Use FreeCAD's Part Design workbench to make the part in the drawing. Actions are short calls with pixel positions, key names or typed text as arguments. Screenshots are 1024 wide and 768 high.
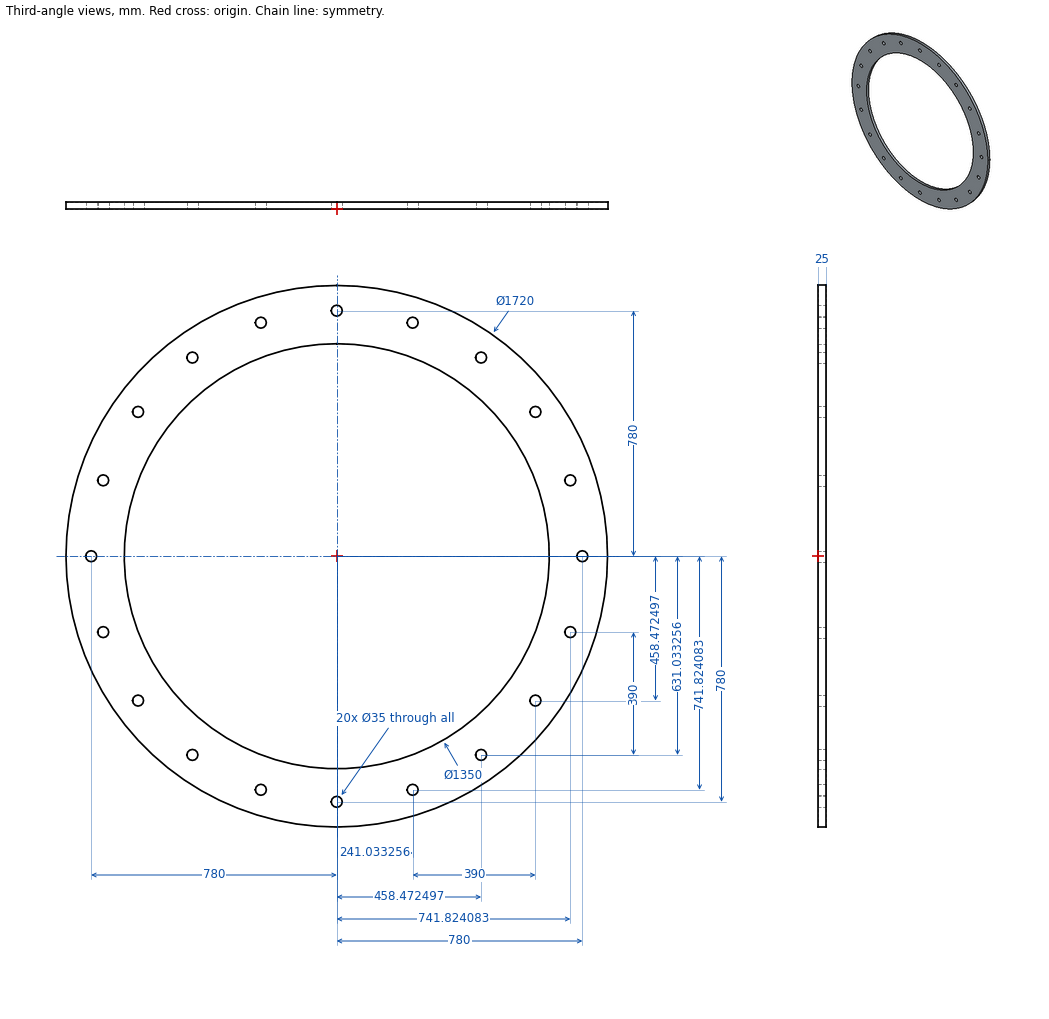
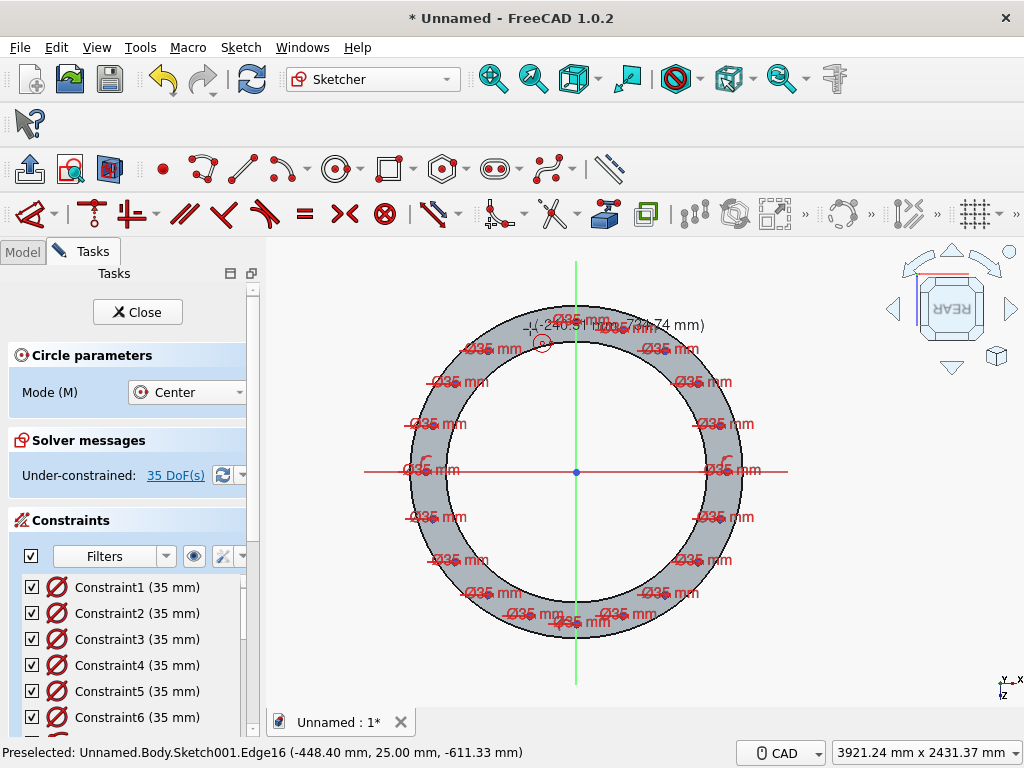
click(530, 329)
move(532, 326)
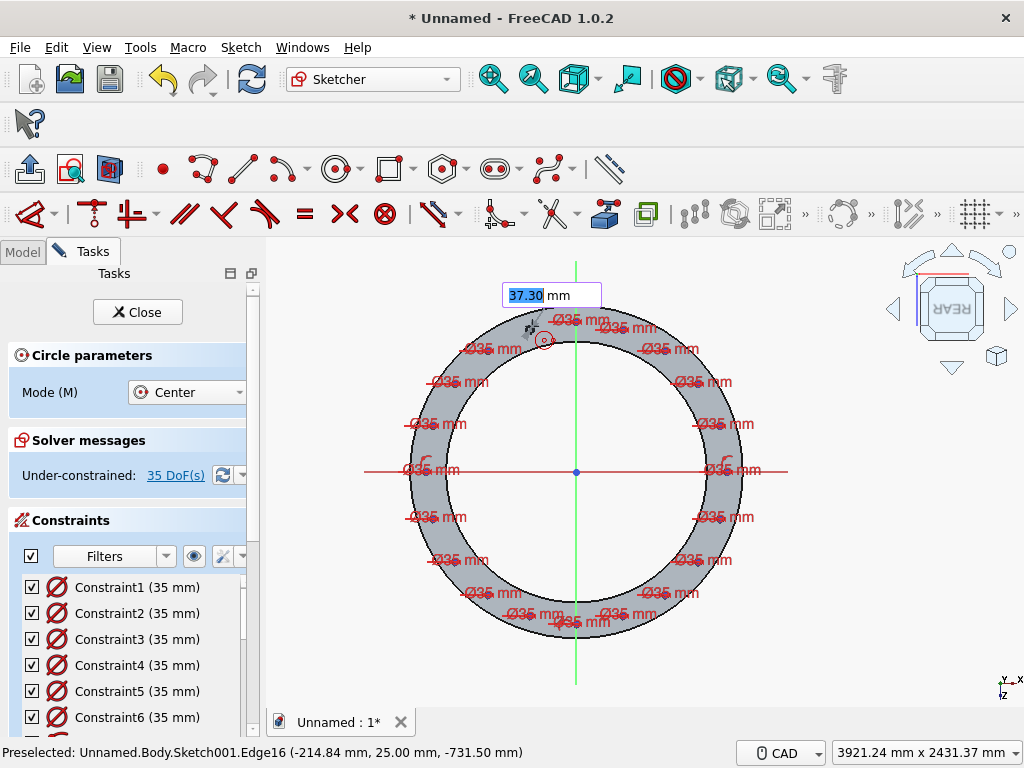
text(35)
key(Return)
key(Escape)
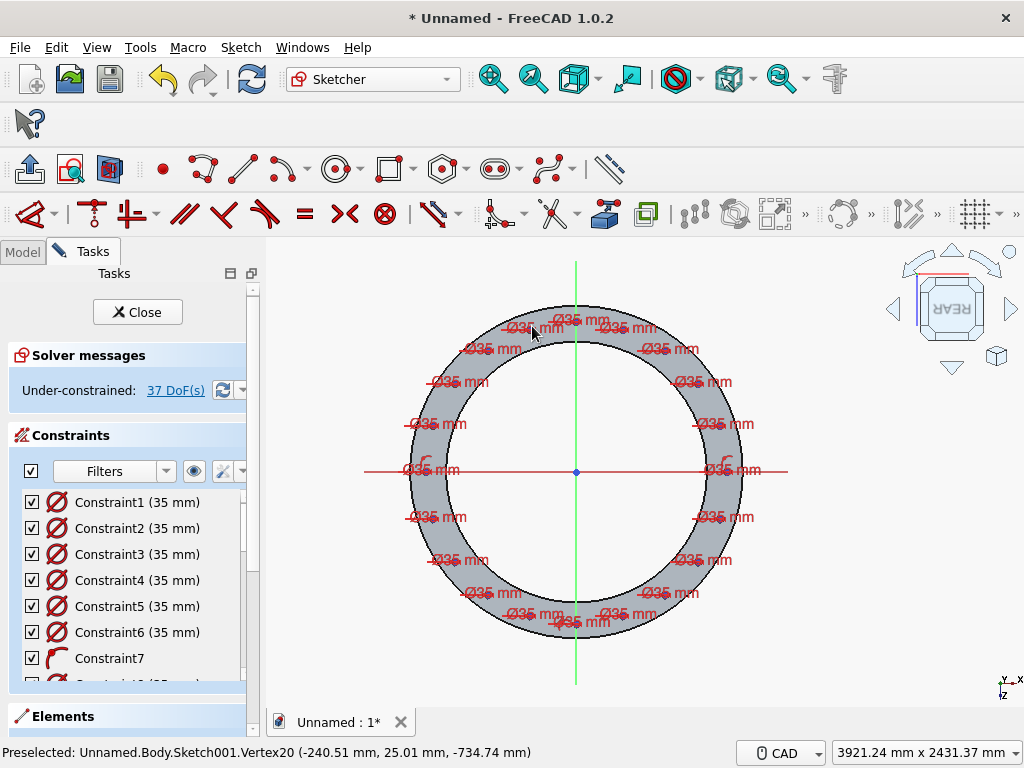
click(576, 322)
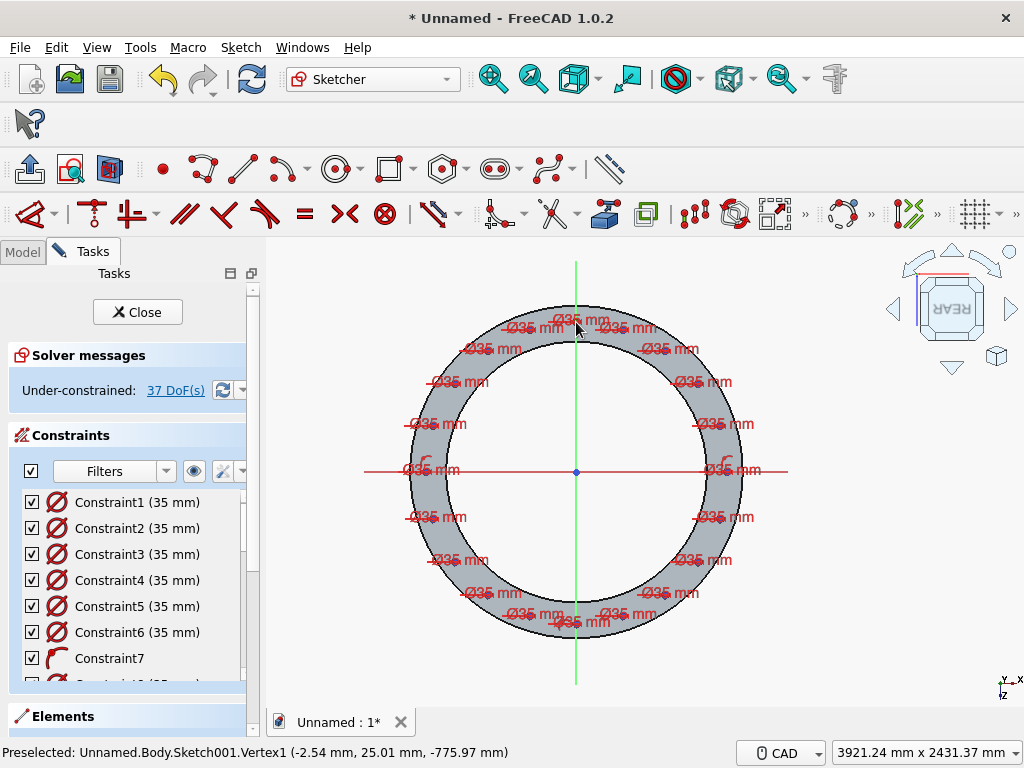
click(576, 590)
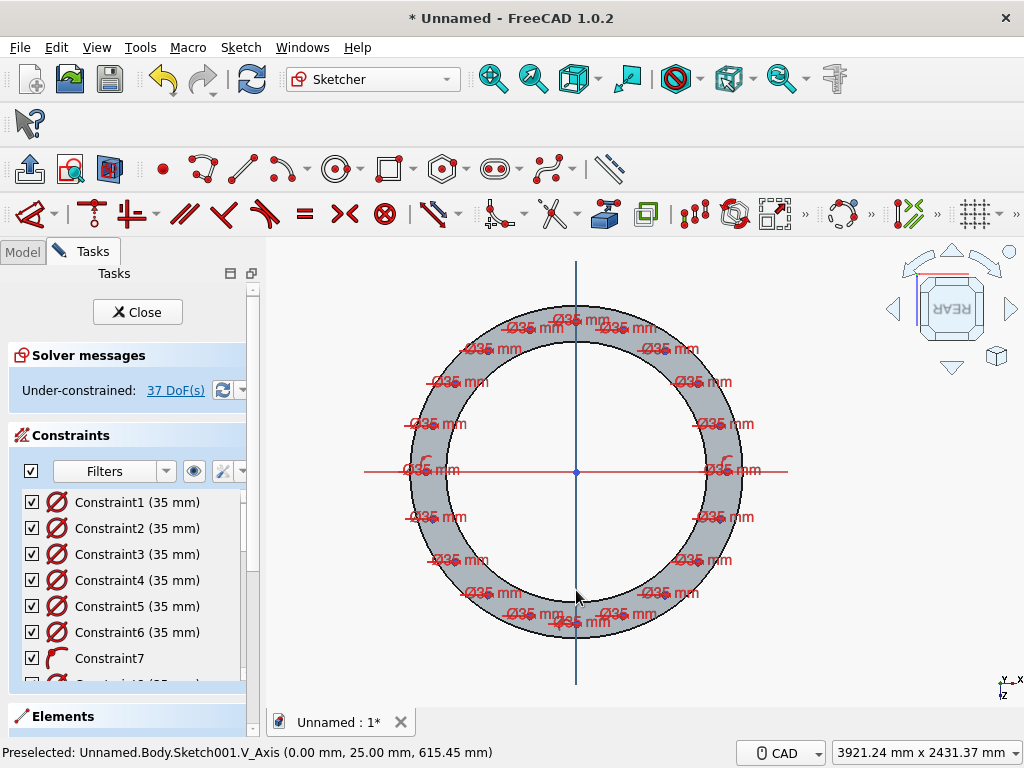
key(c)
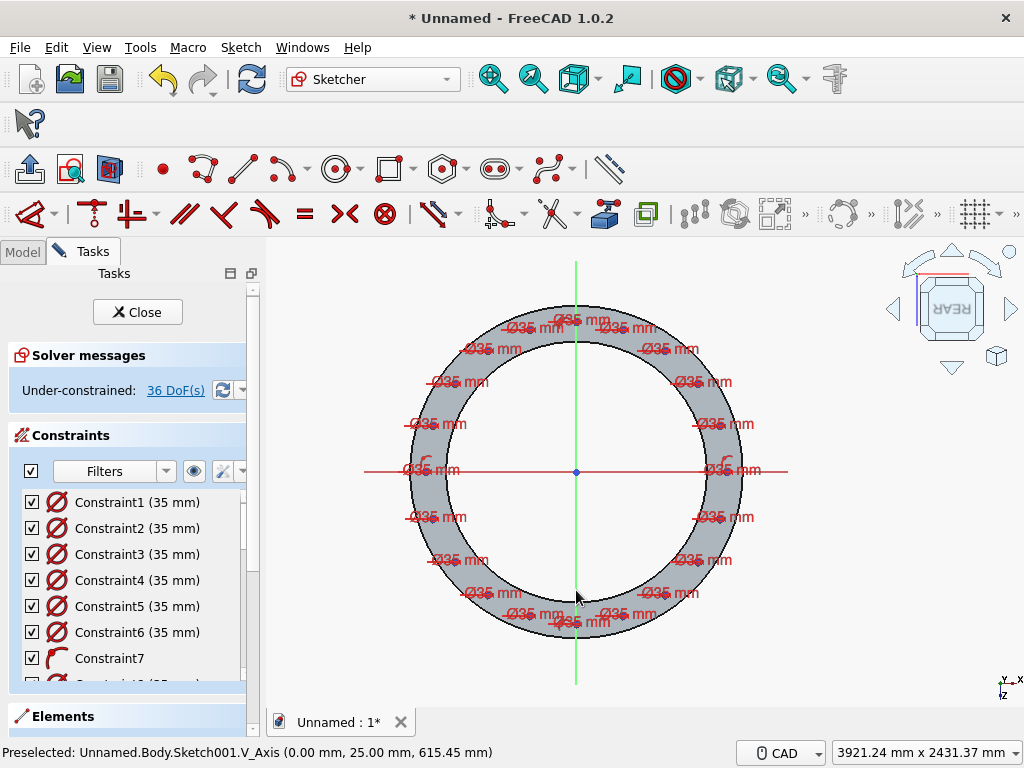
click(720, 426)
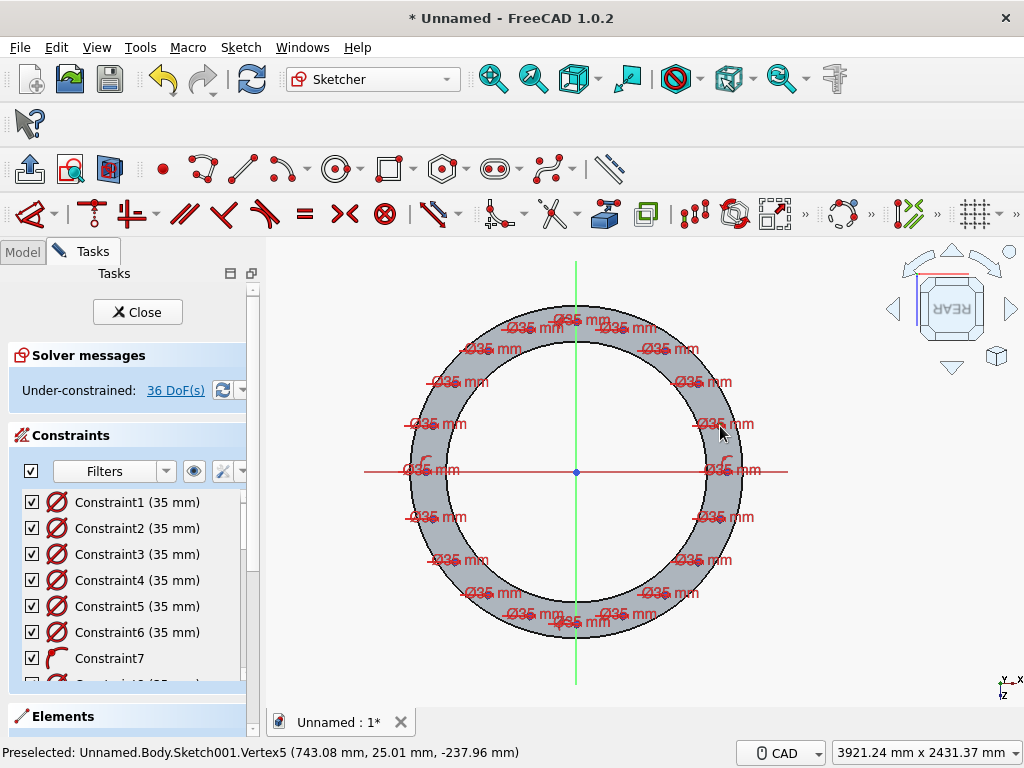
click(720, 519)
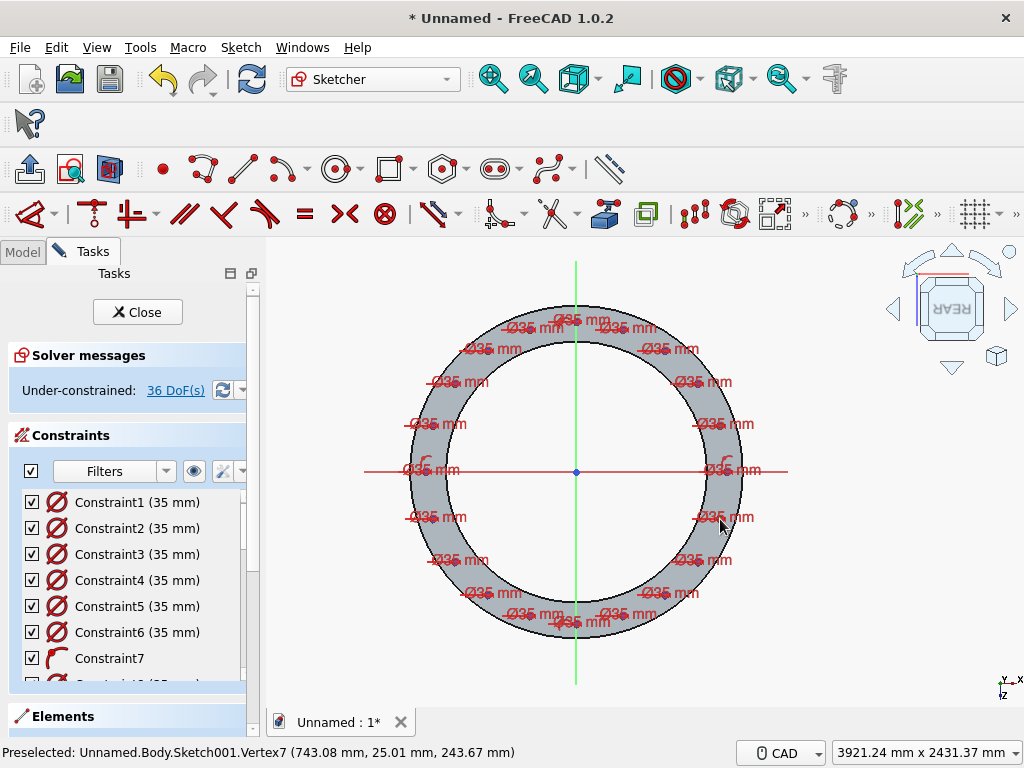
click(375, 472)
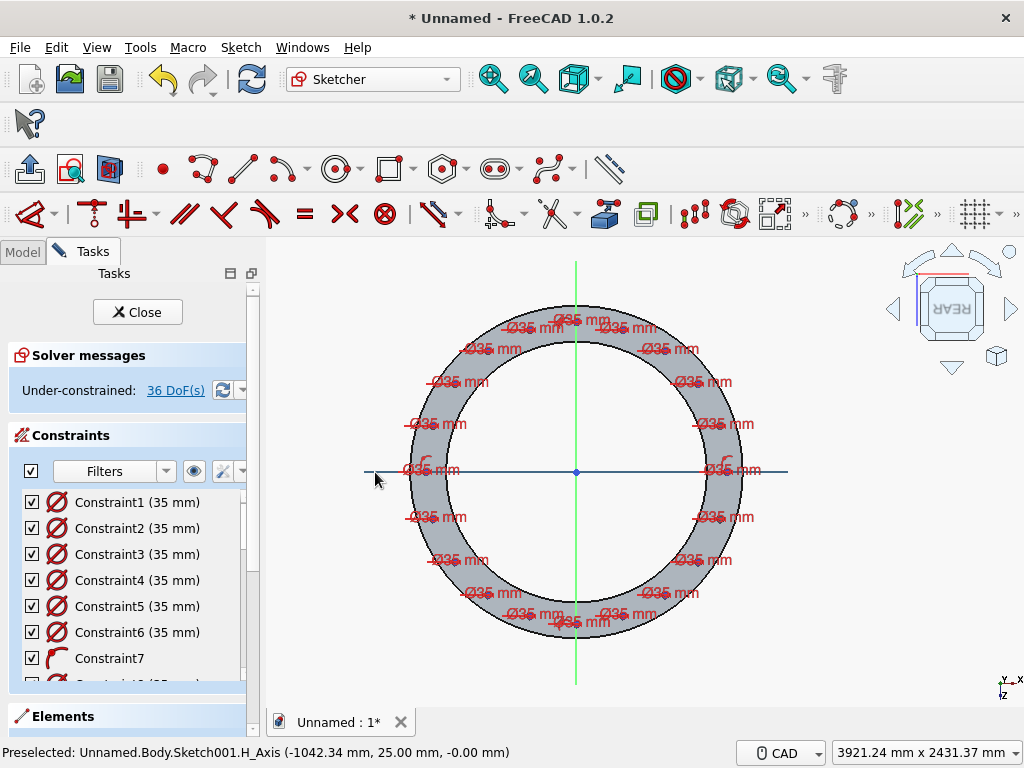
click(346, 214)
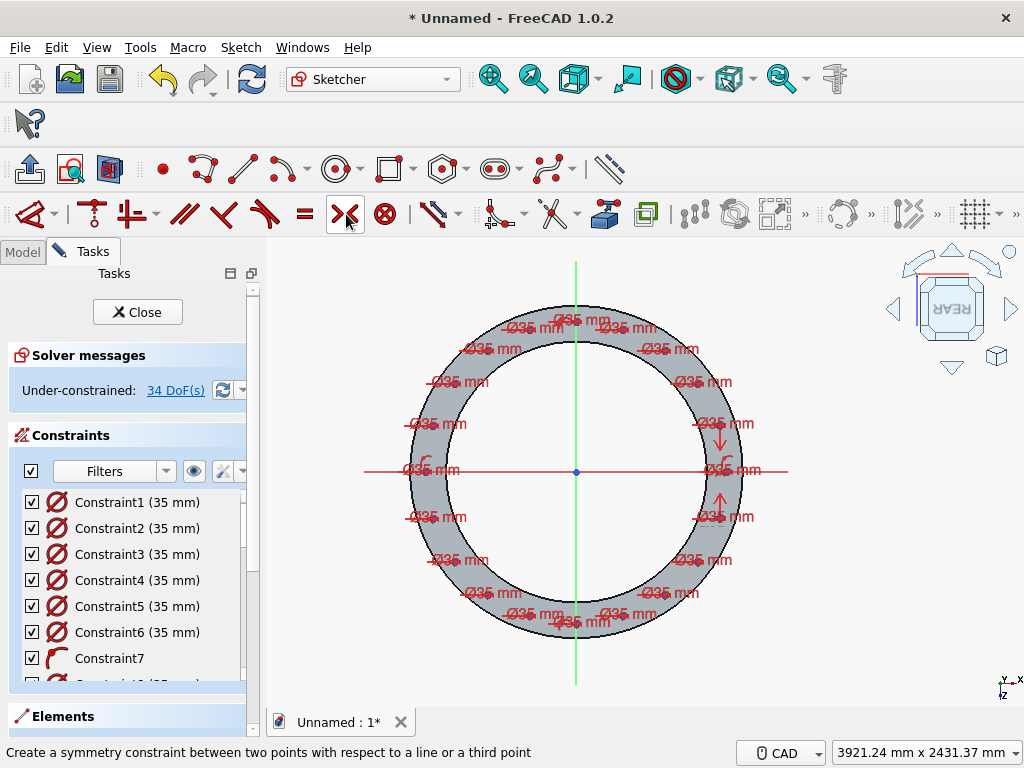
click(698, 384)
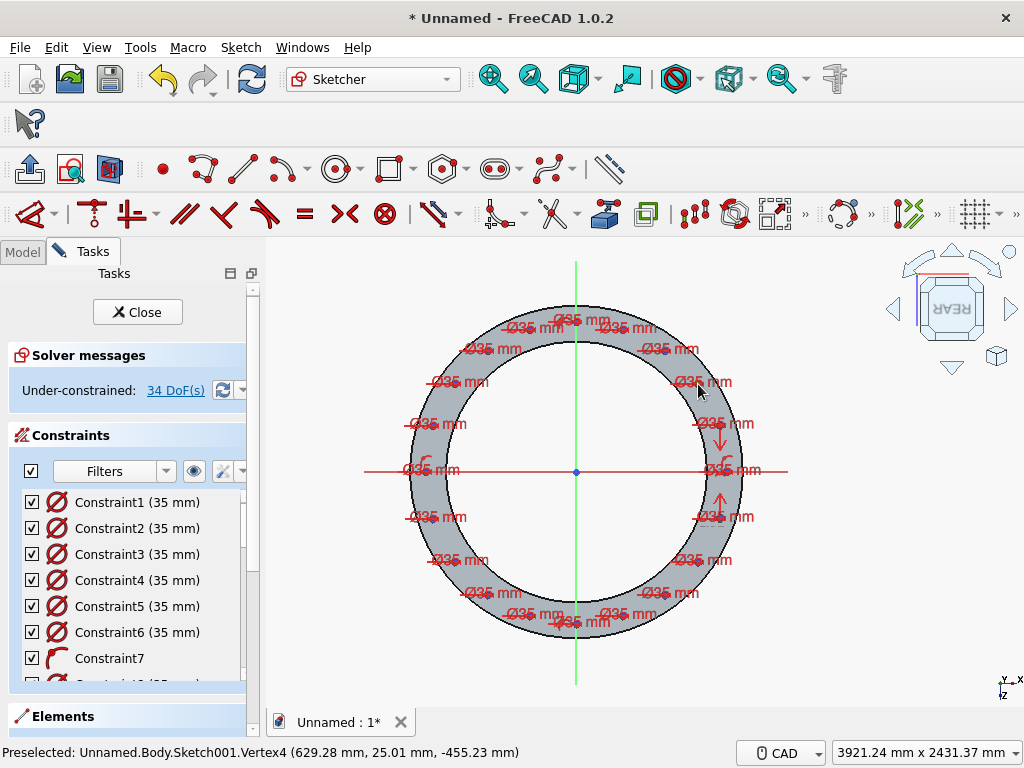
click(698, 562)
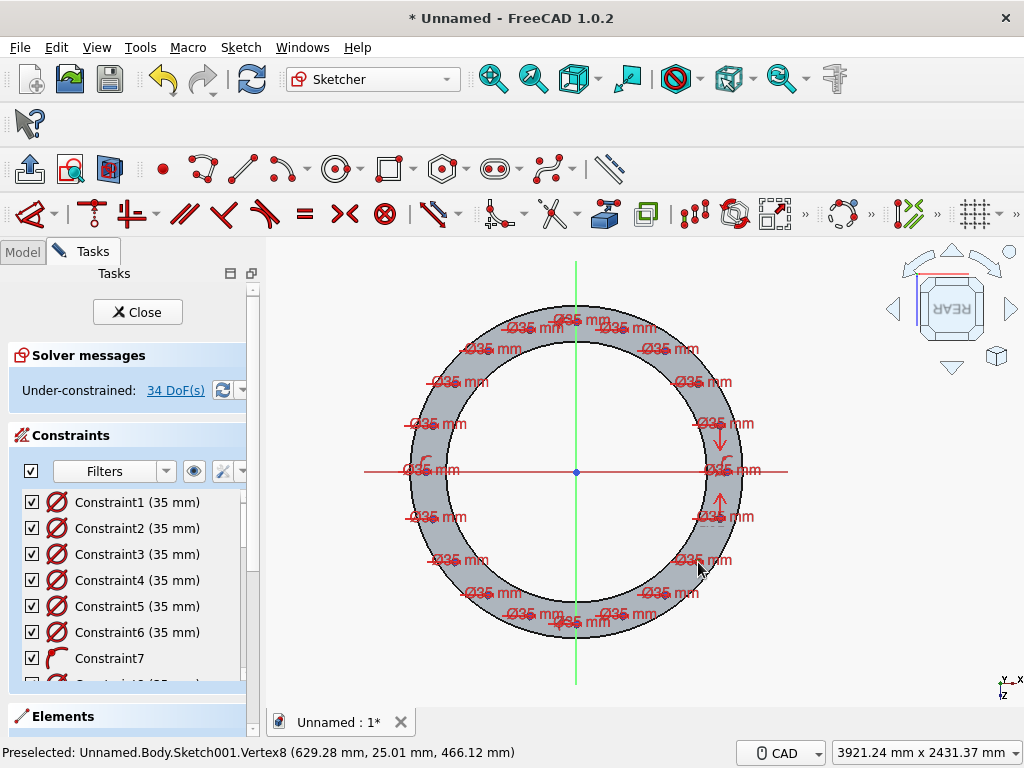
click(375, 472)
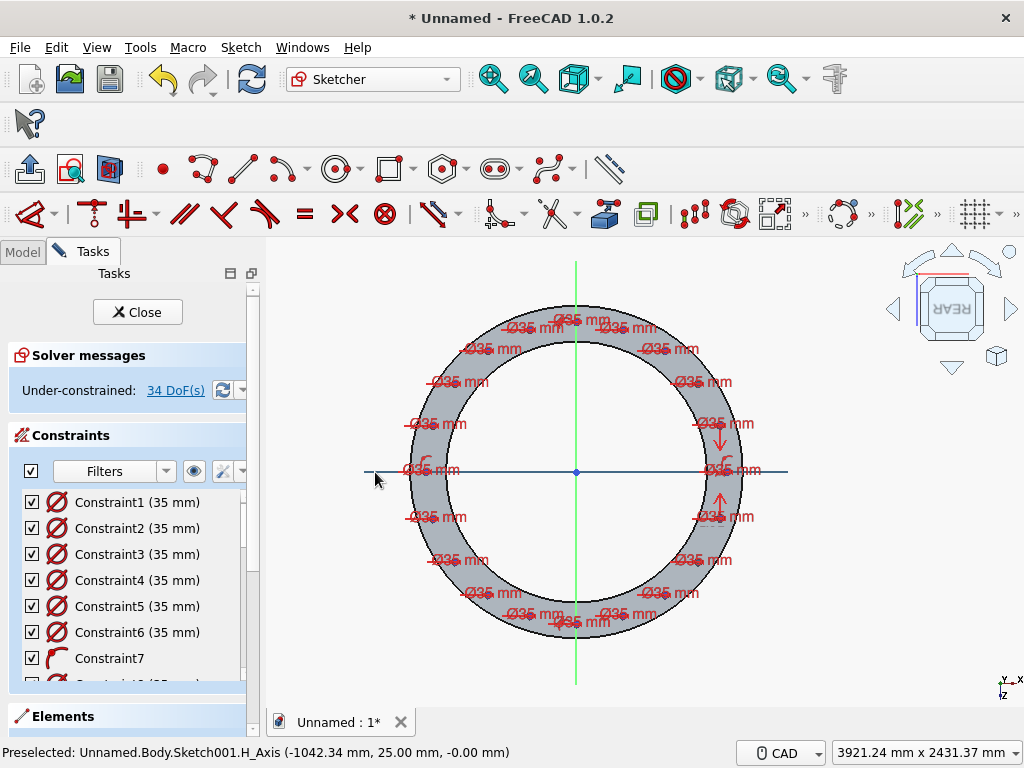
key(s)